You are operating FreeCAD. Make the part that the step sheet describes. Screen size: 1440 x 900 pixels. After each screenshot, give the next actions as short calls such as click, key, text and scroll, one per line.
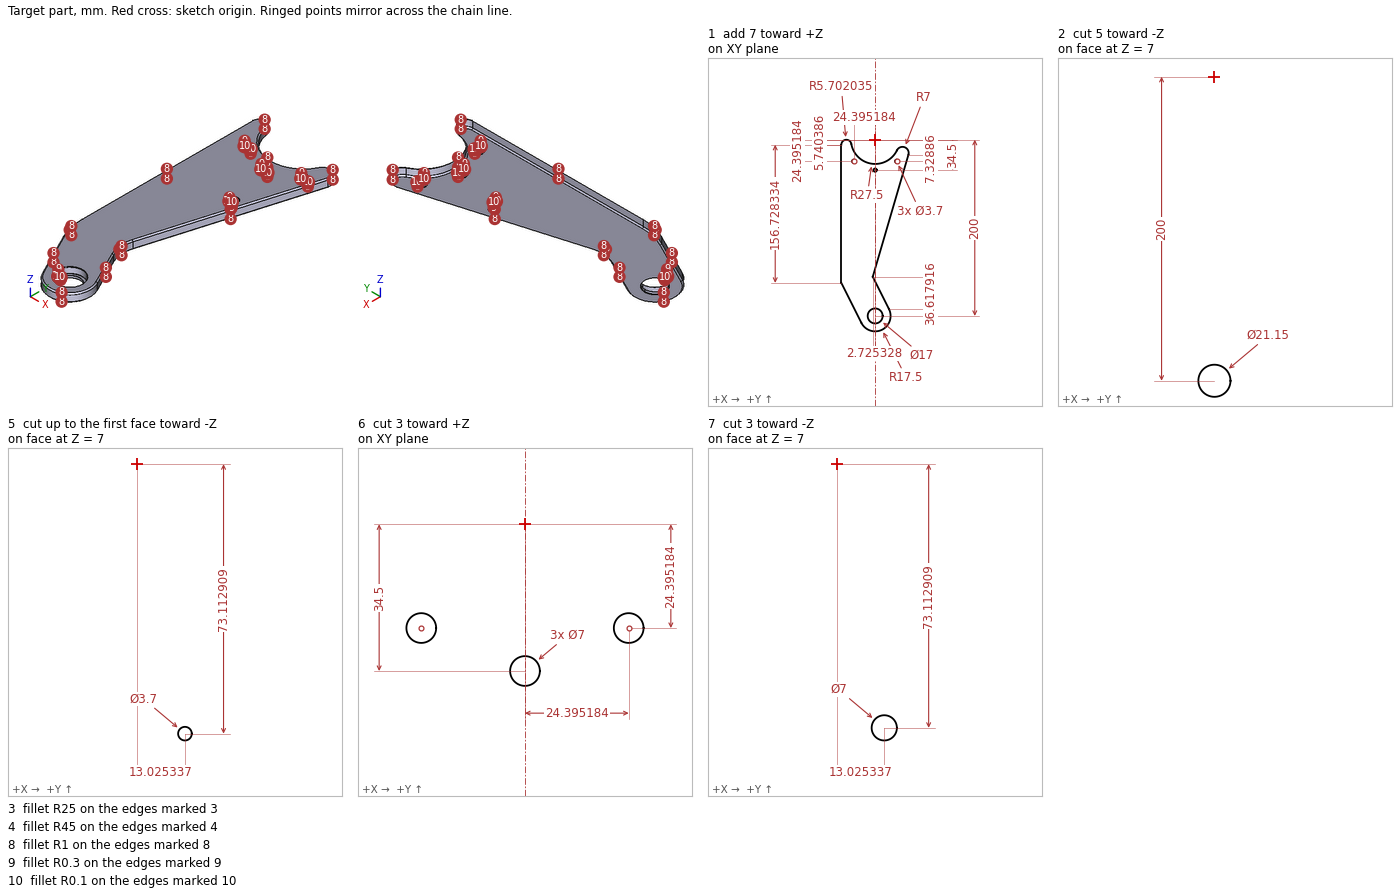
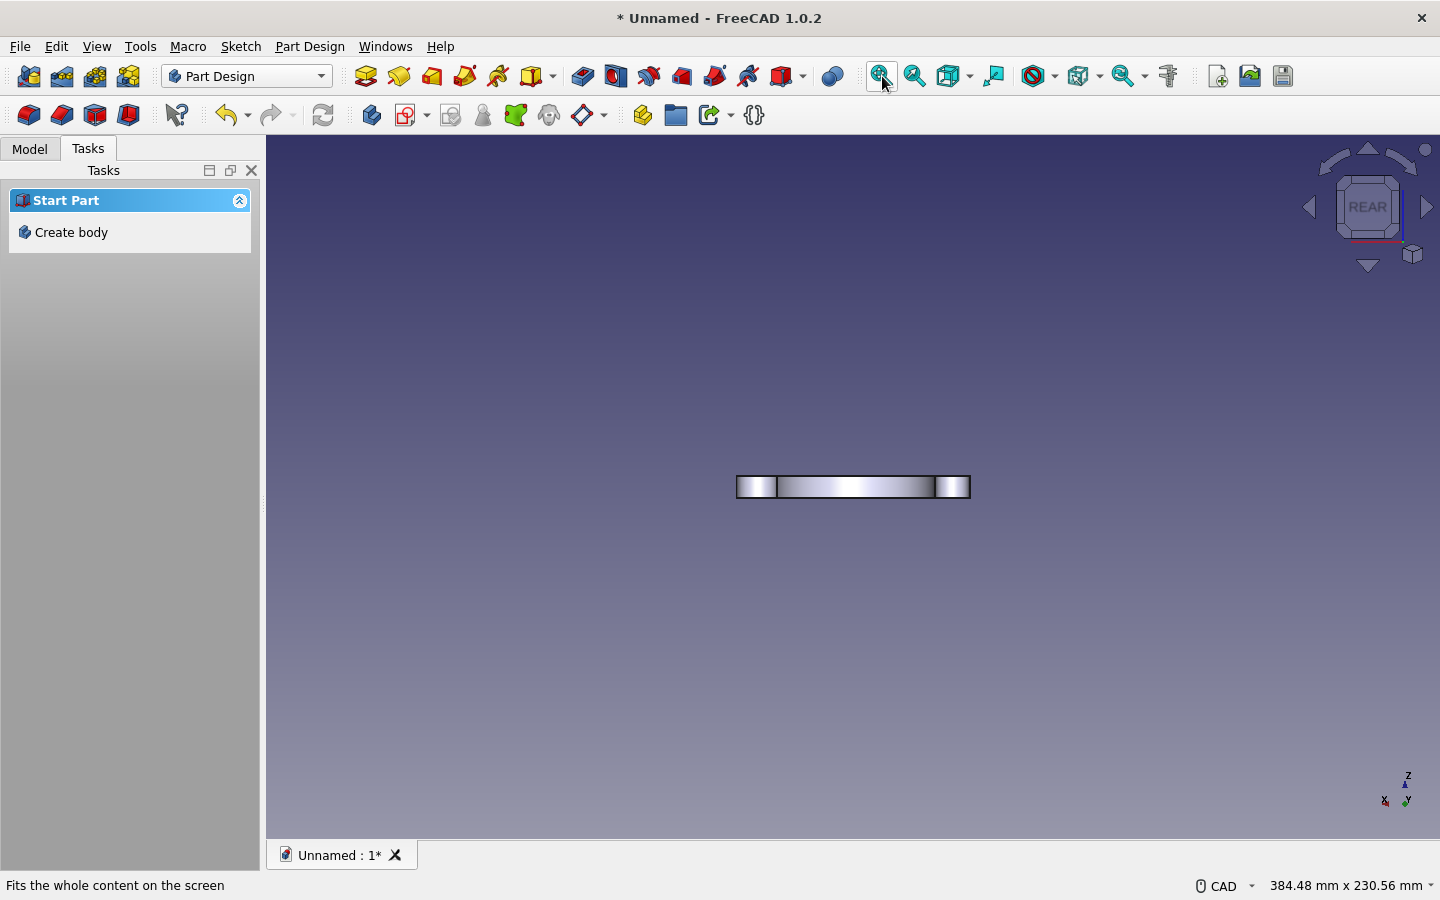
scroll(861, 486, up, 4)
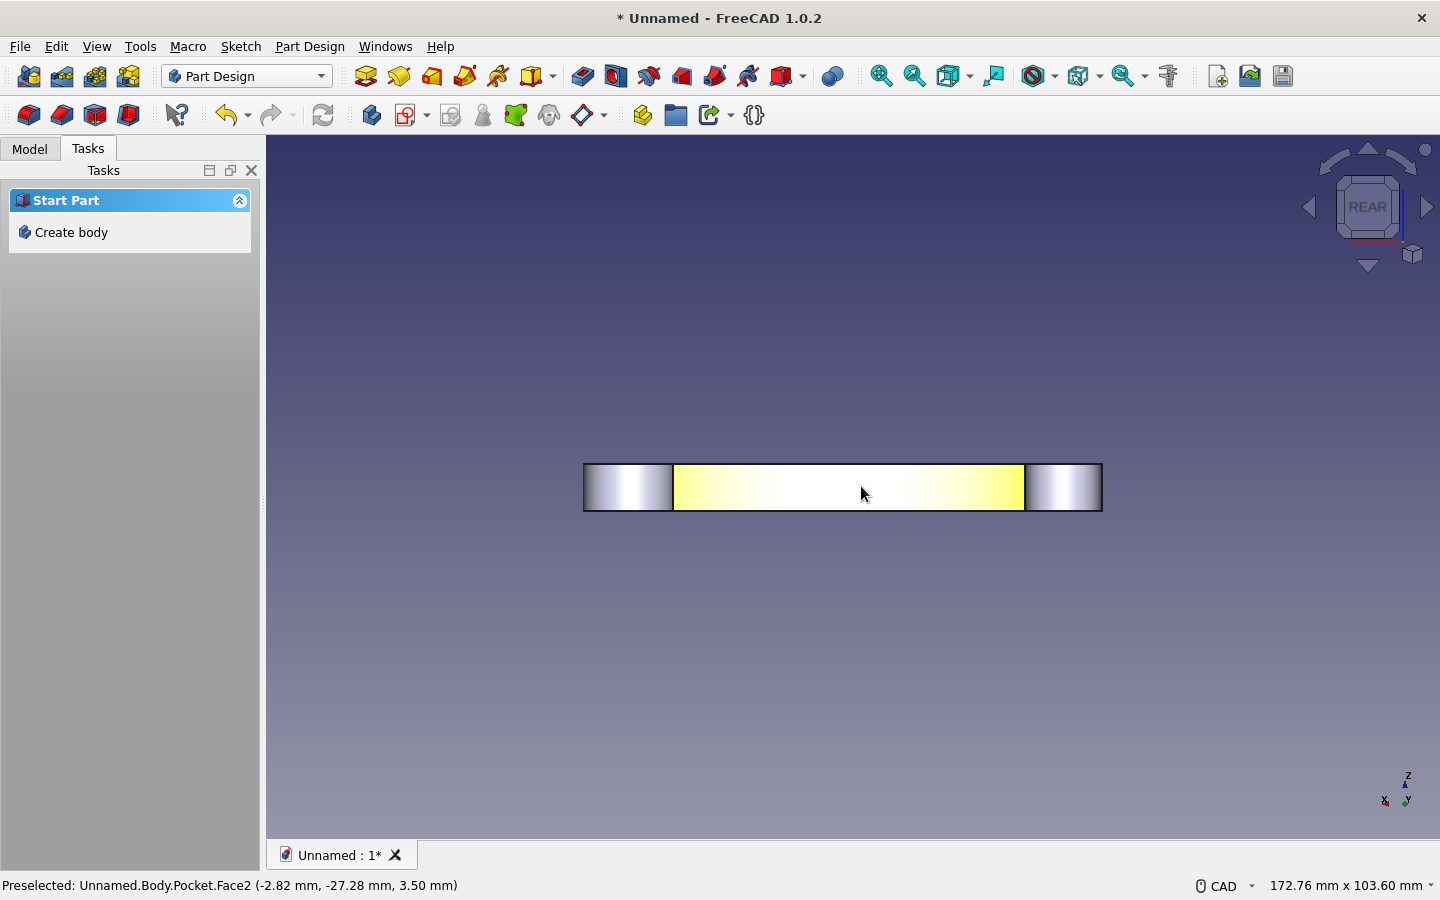
key(v)
key(f)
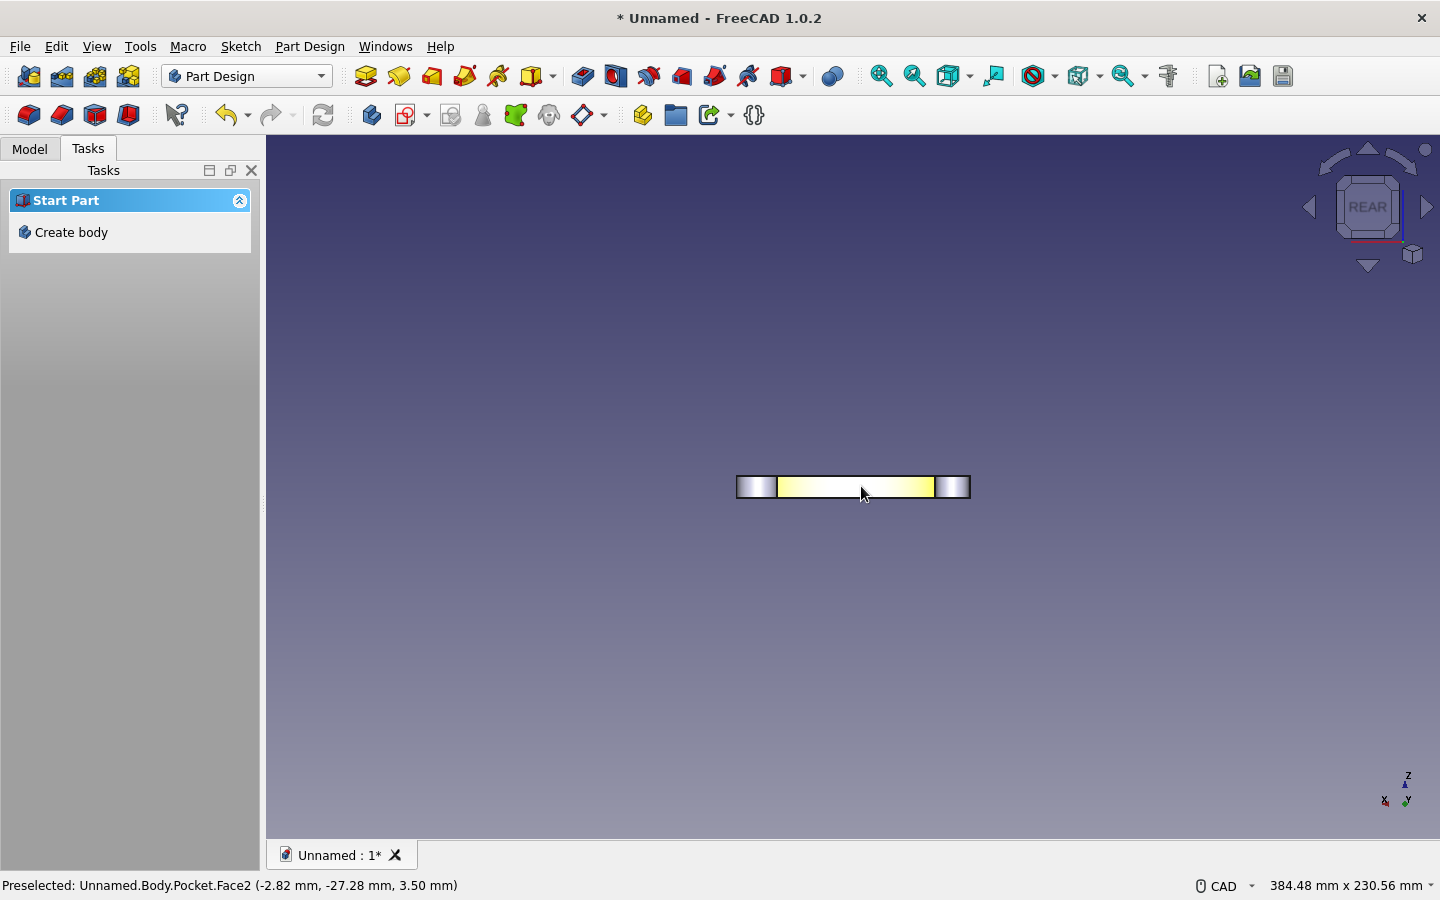
key(6)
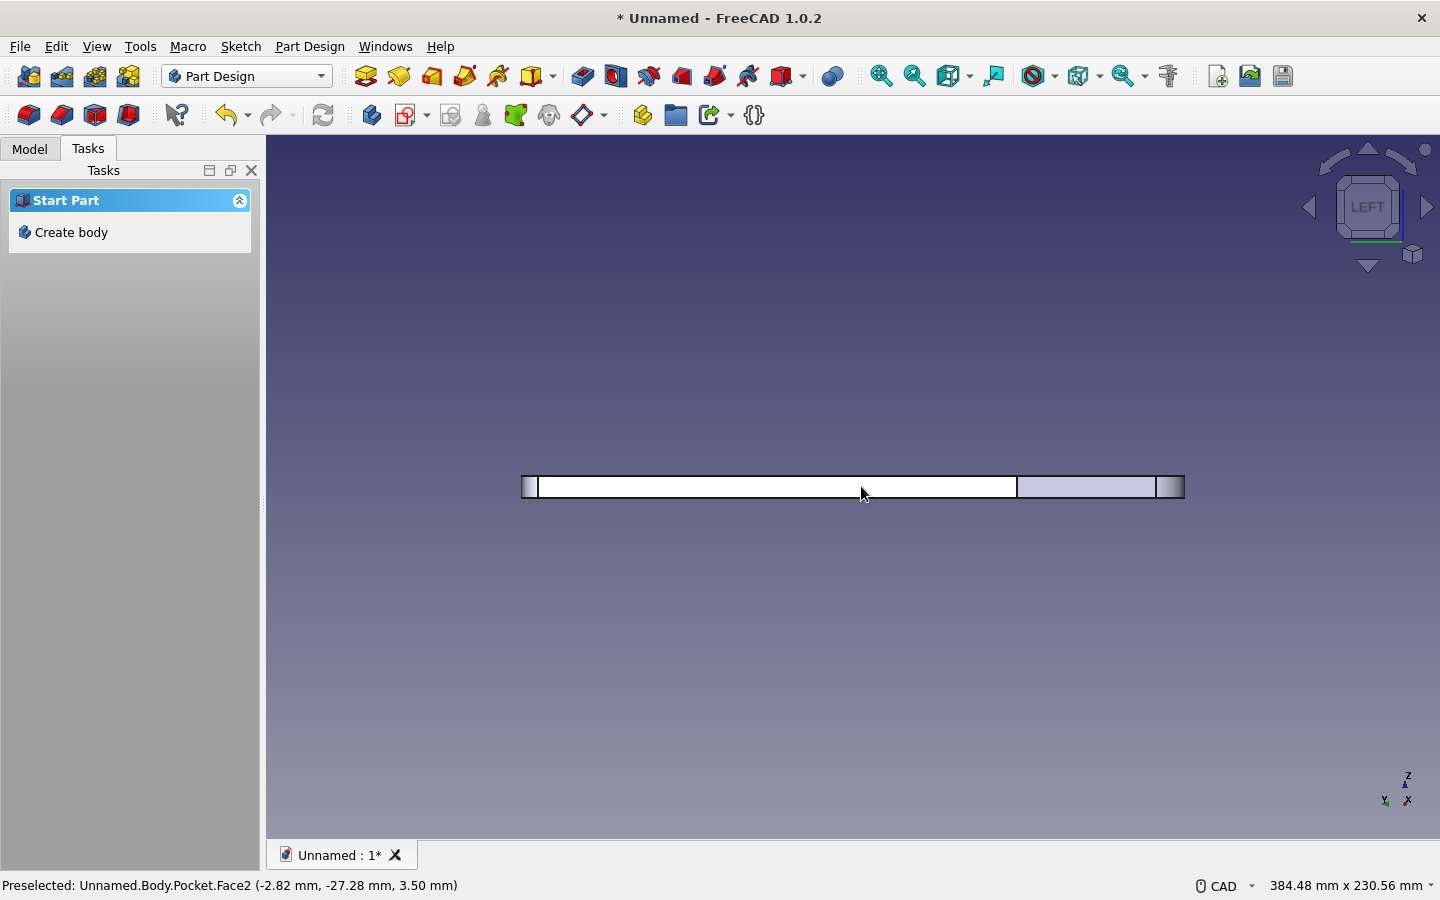
scroll(996, 486, up, 4)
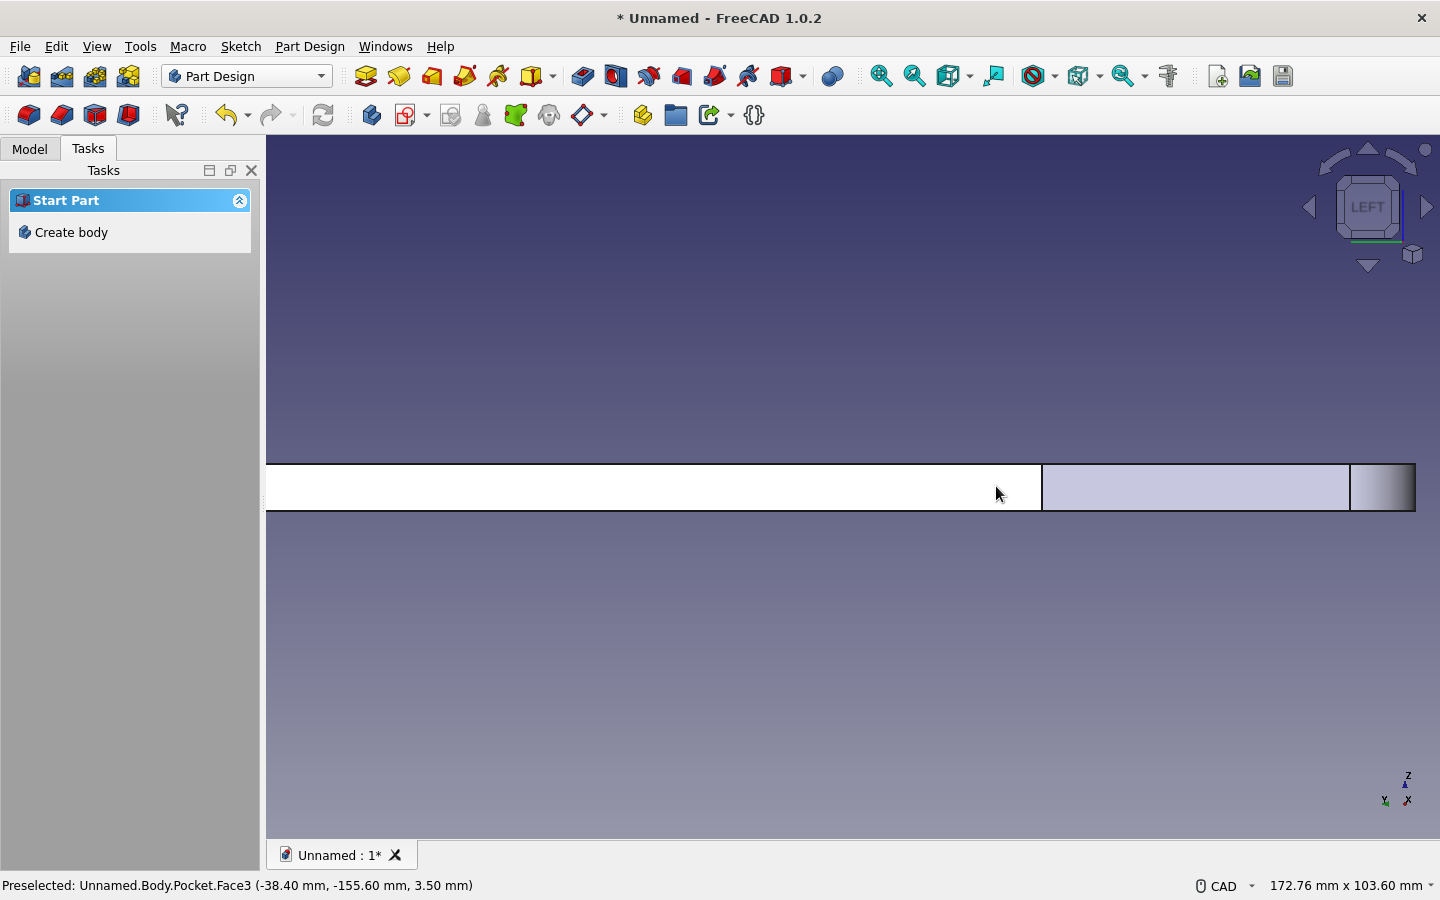
click(882, 76)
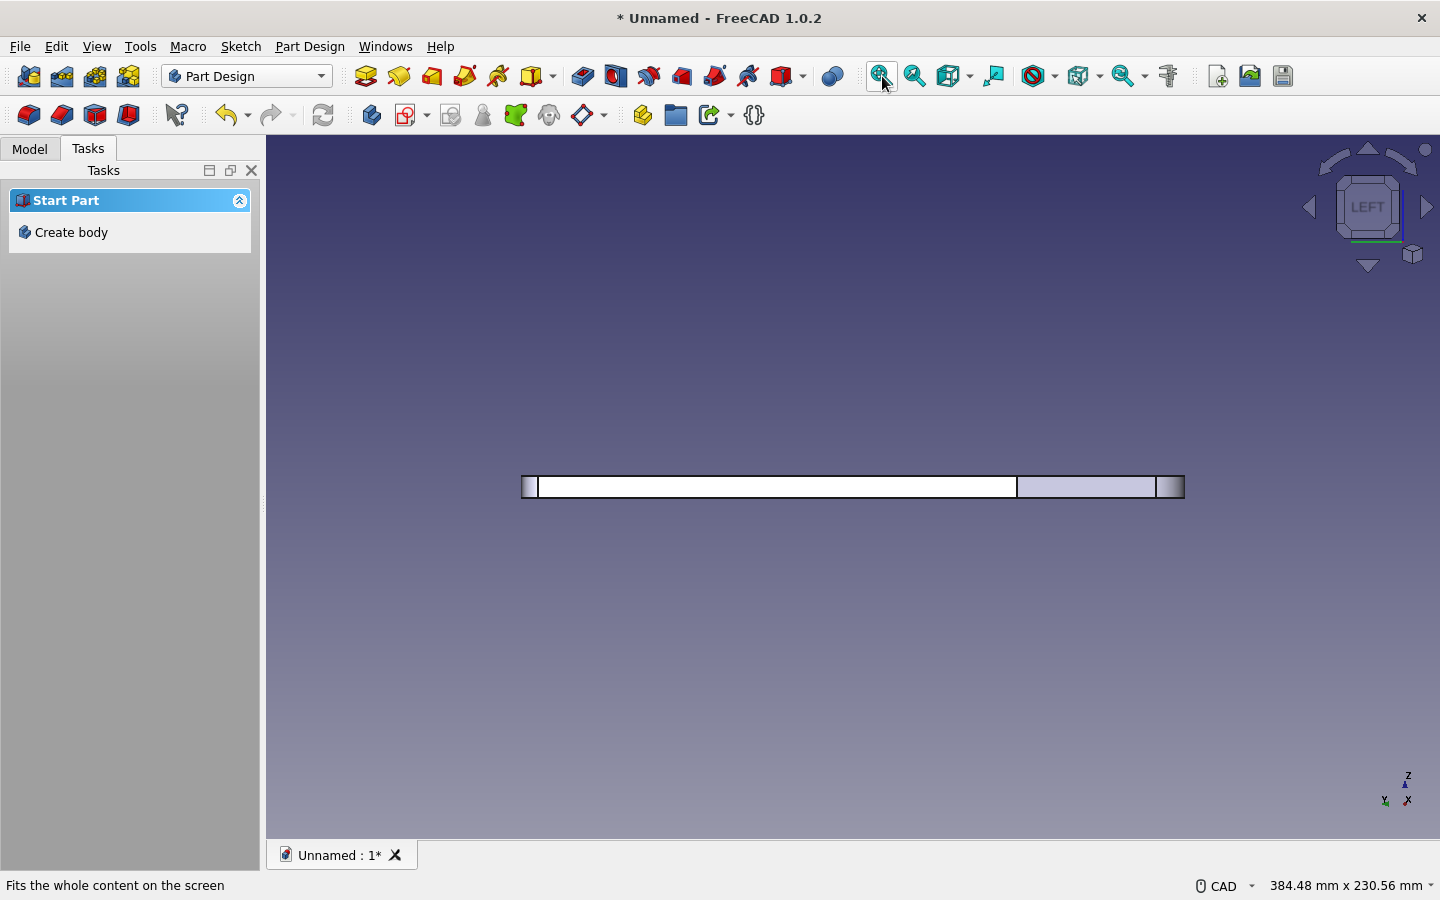
key(v)
key(3)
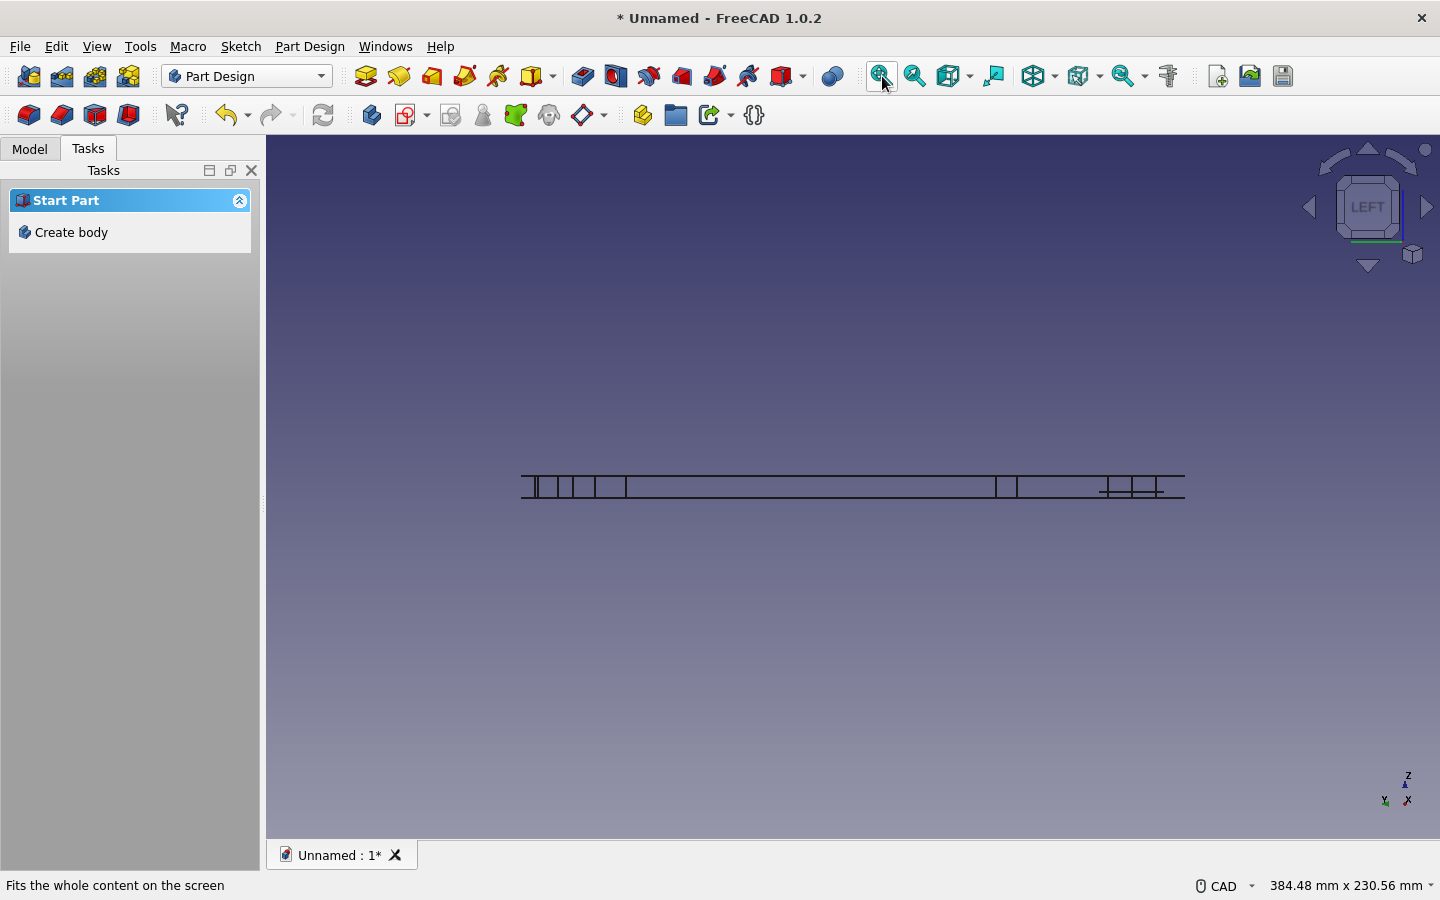
key(0)